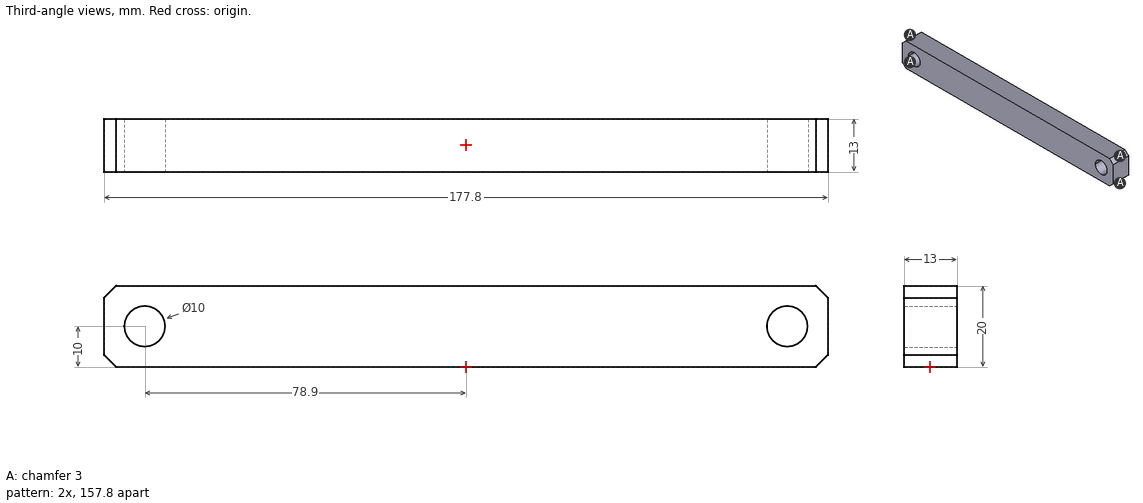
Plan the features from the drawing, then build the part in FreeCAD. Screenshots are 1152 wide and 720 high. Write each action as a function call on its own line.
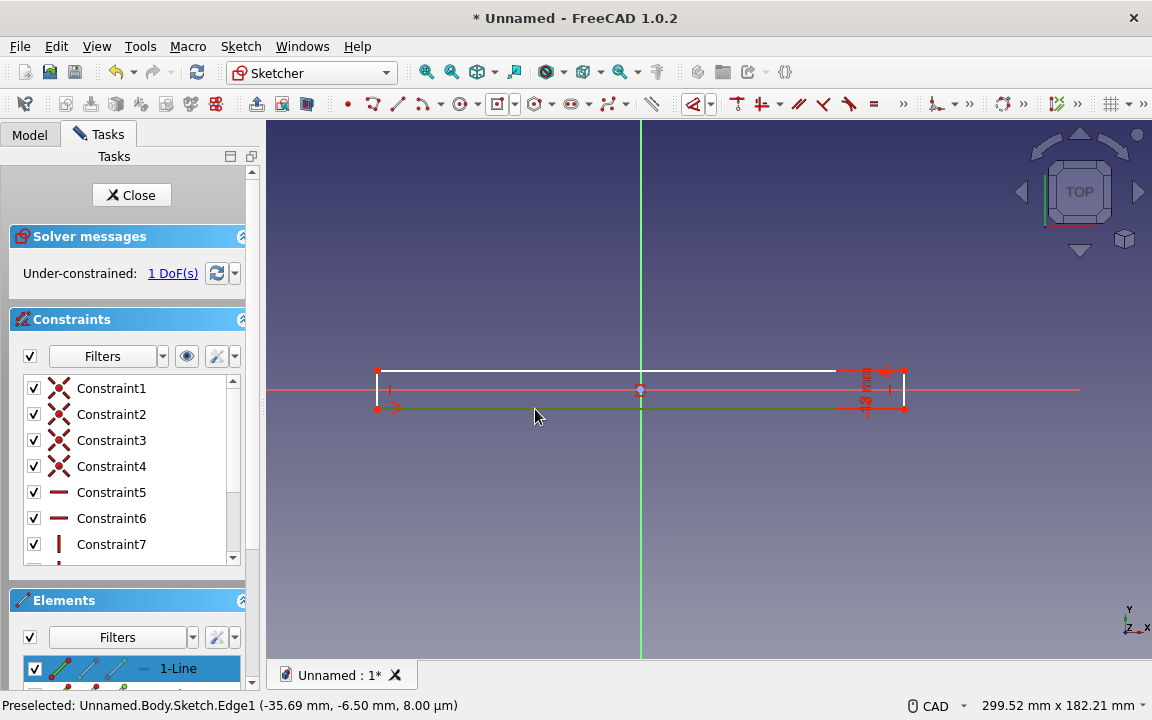
click(710, 104)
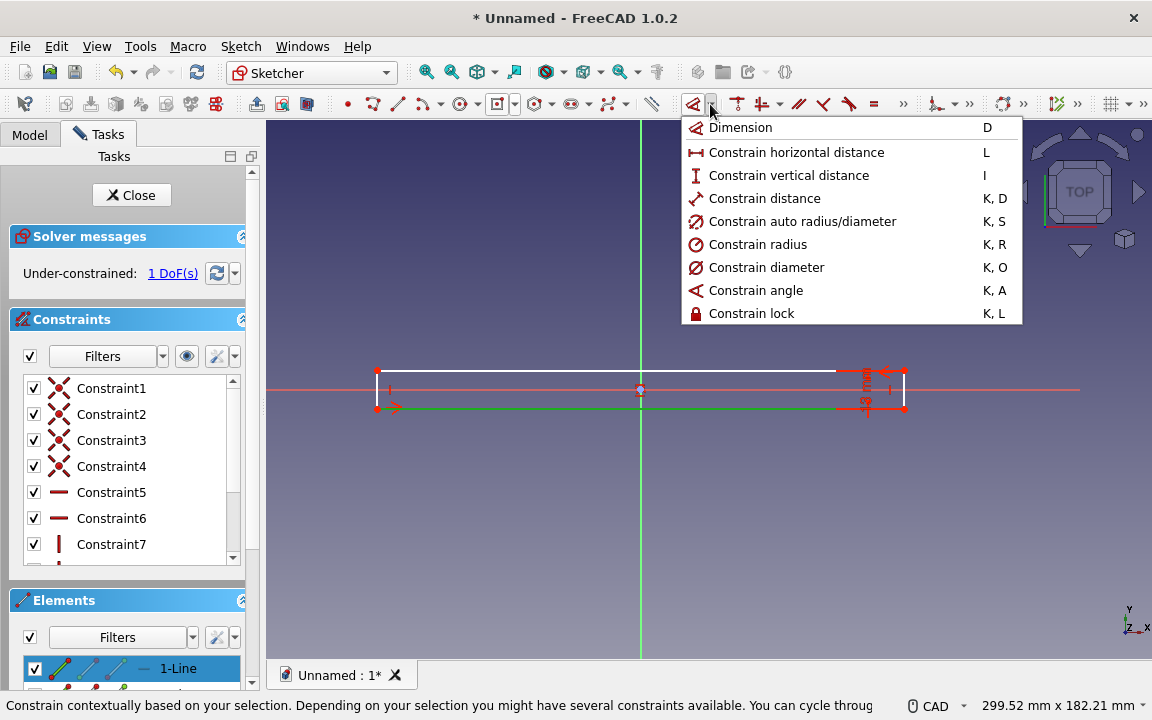
click(852, 152)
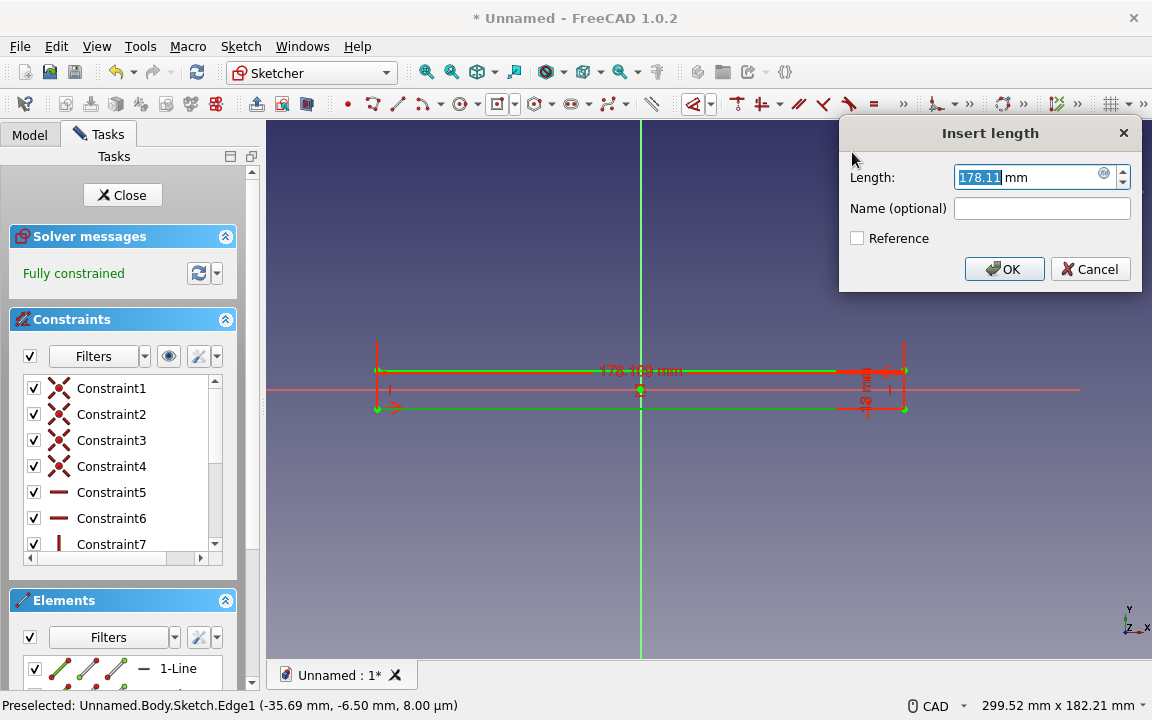
text(177.8)
key(Return)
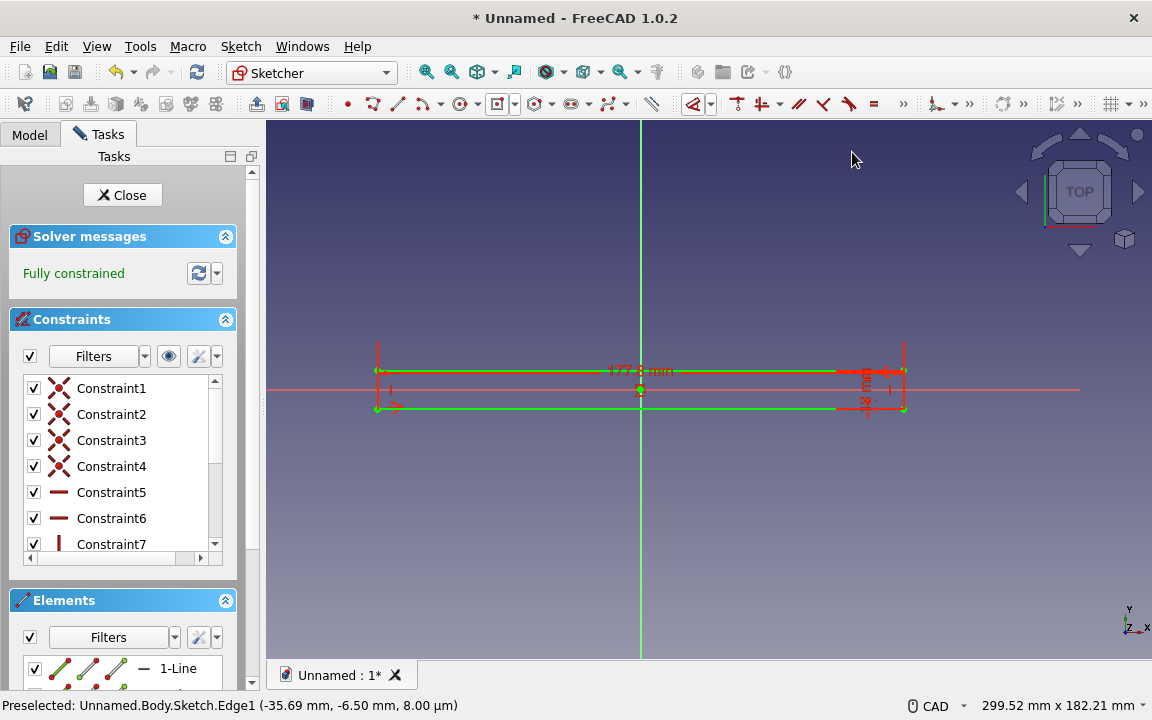
click(123, 195)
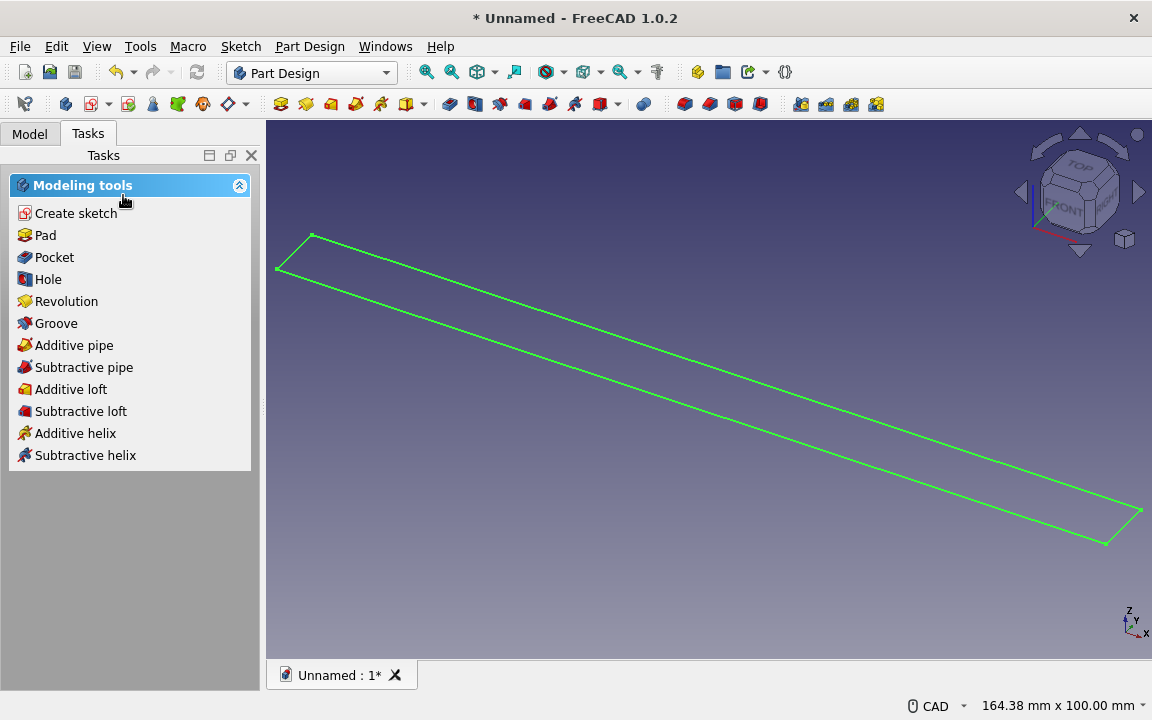
click(281, 104)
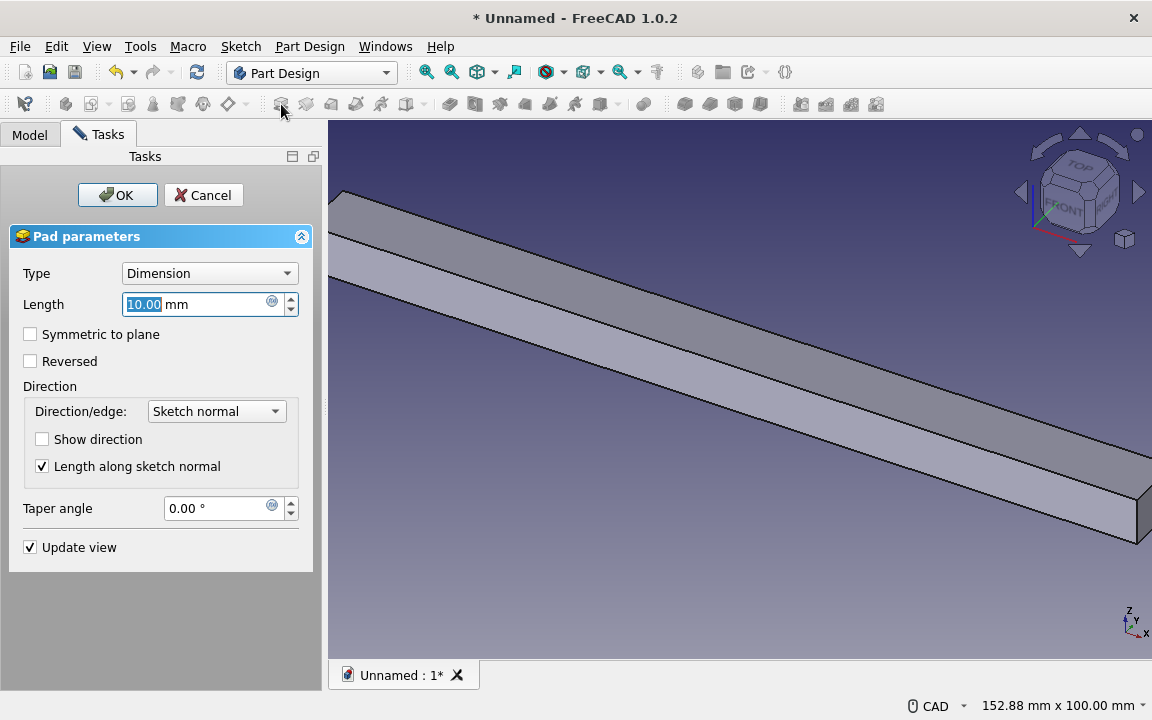
text(20)
key(Tab)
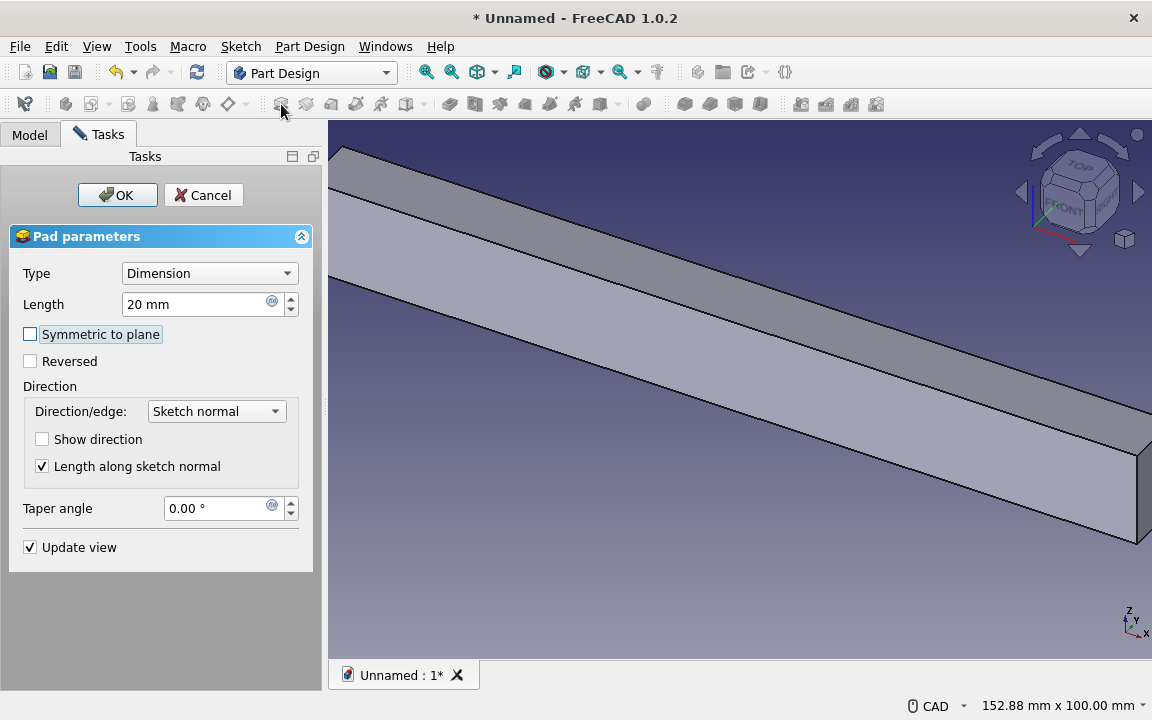
click(118, 195)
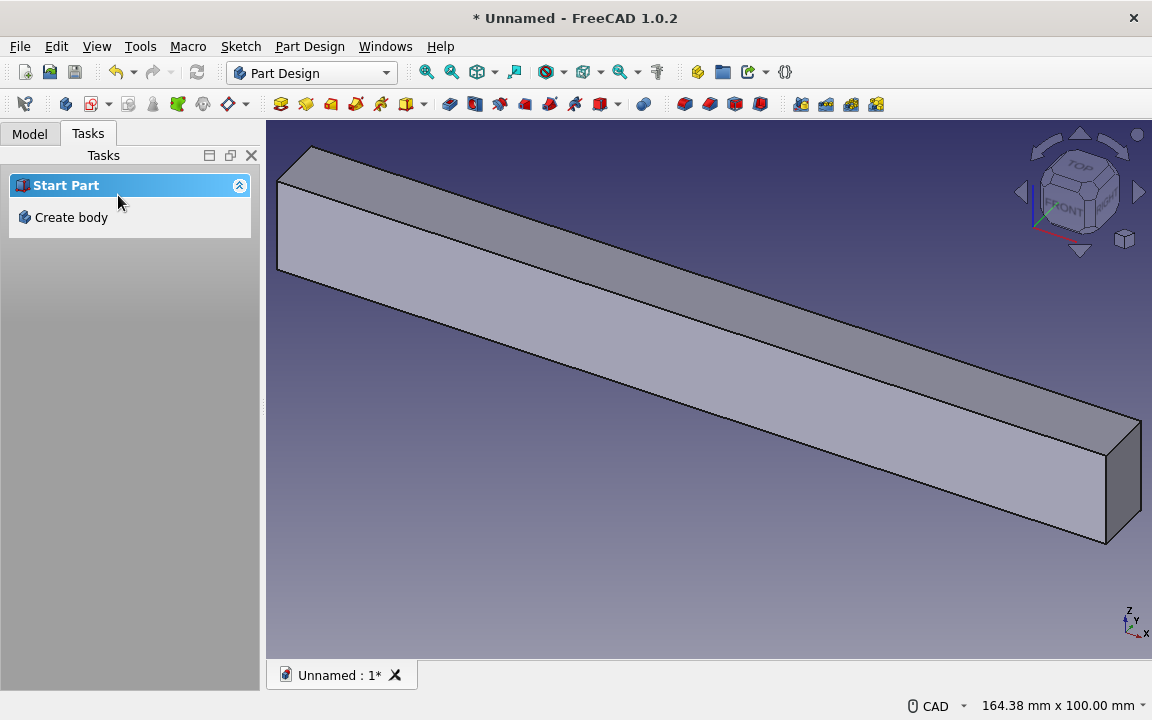
key(0)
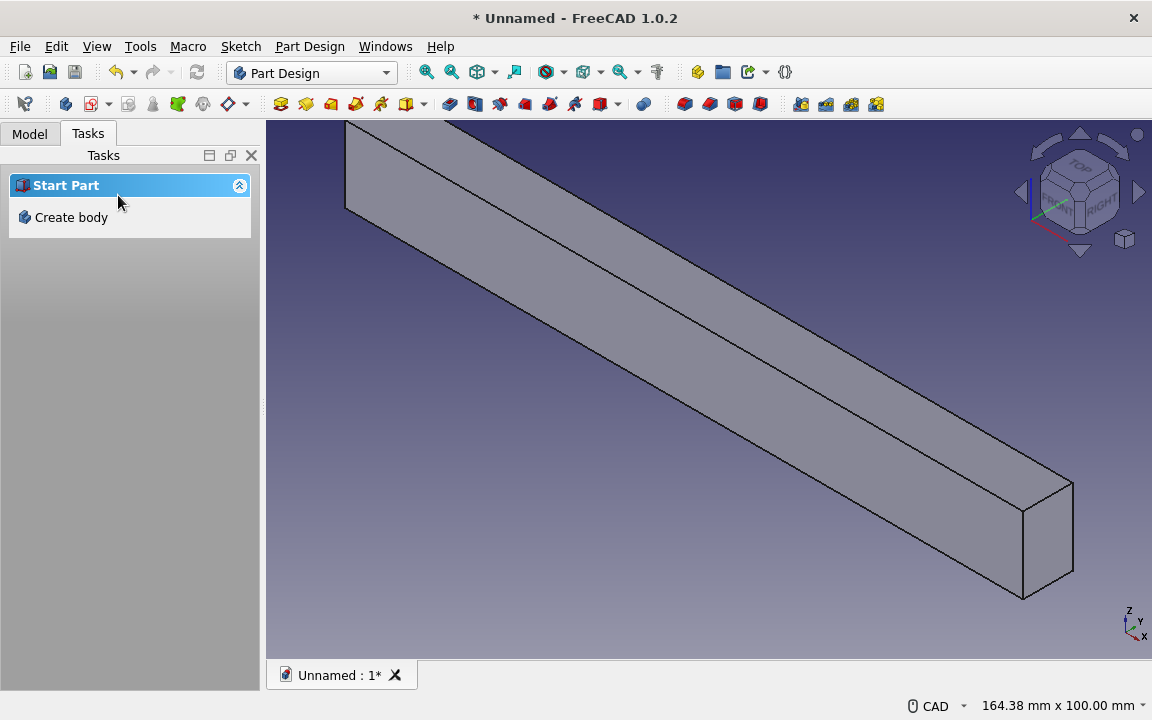
click(427, 72)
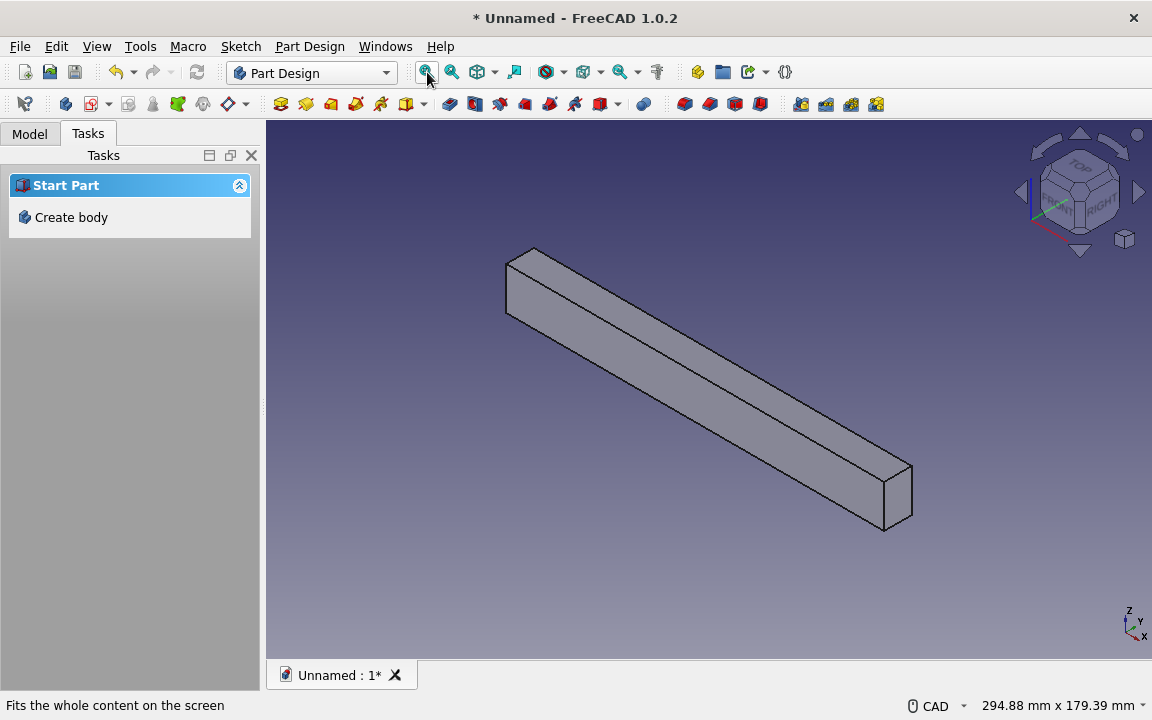
click(898, 473)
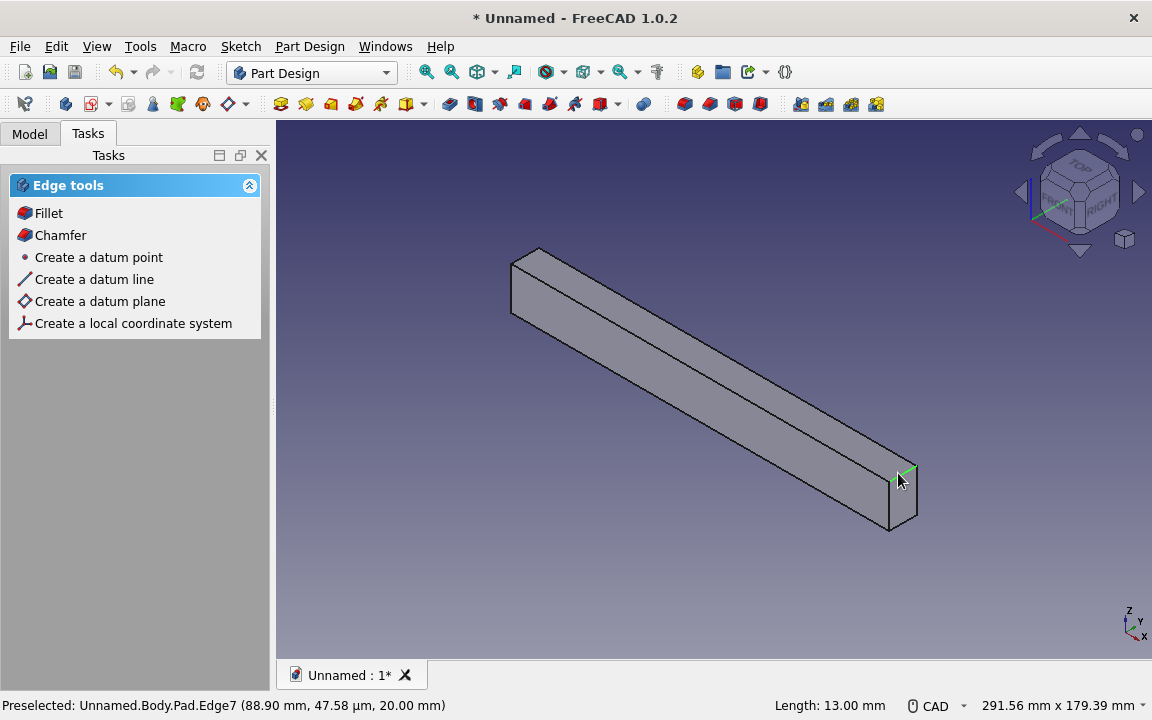
key(2)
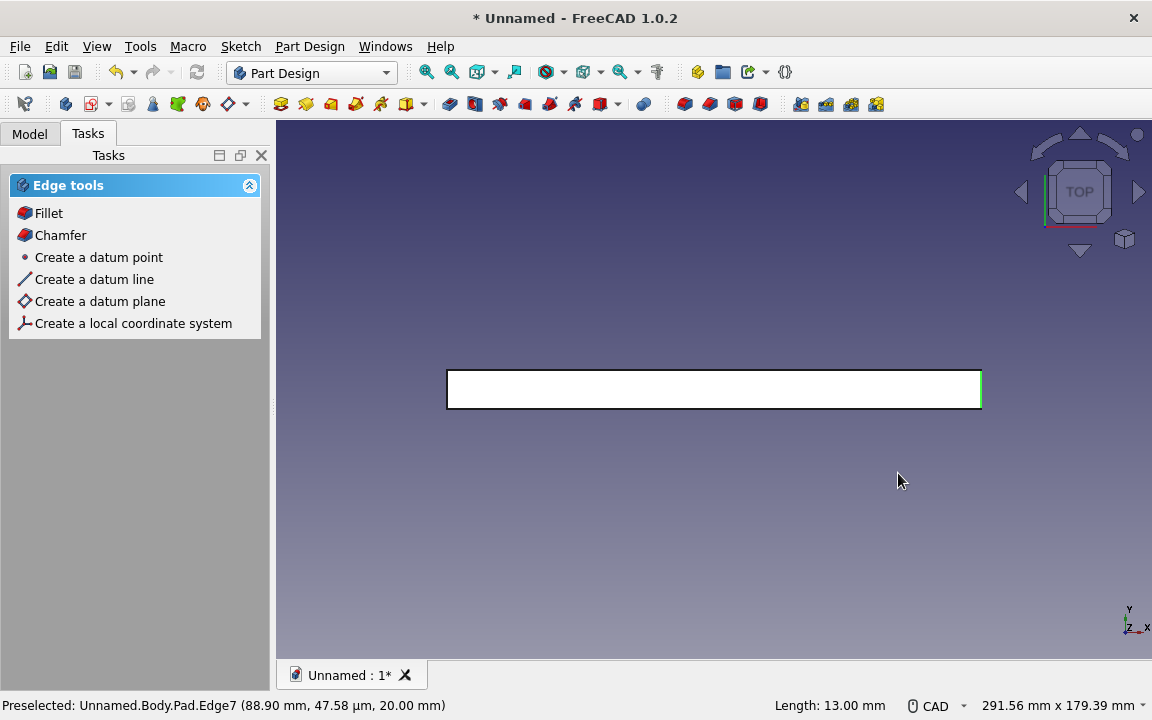
click(447, 388, ctrl)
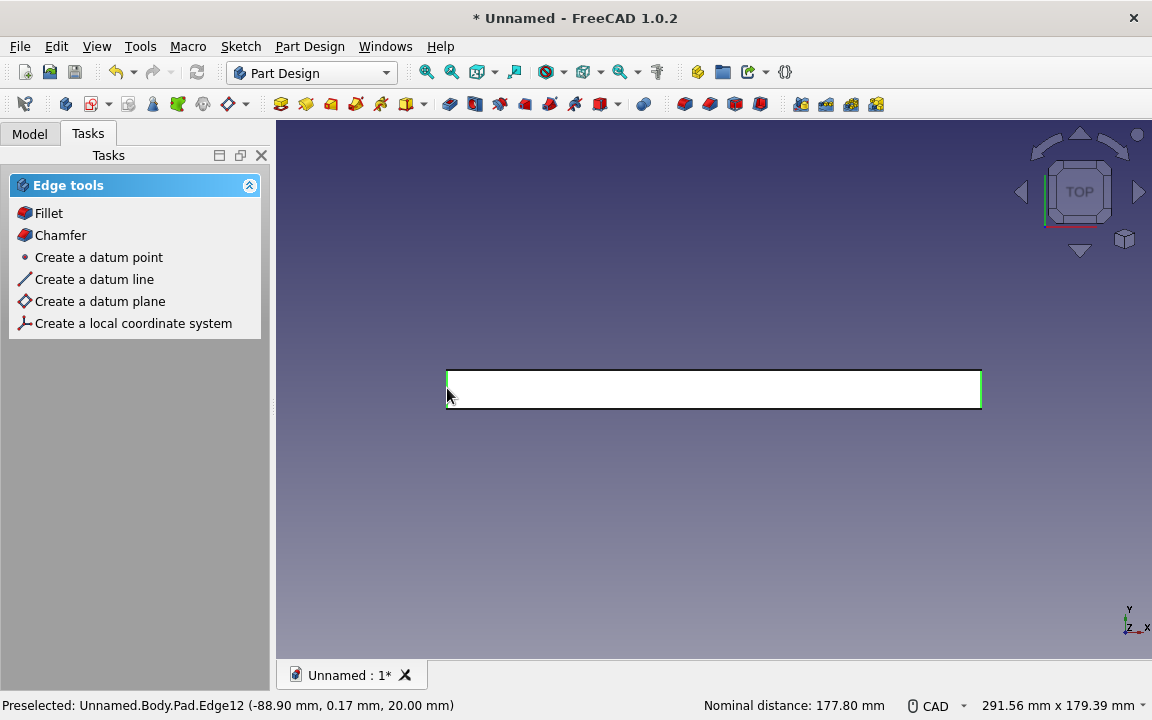
key(1)